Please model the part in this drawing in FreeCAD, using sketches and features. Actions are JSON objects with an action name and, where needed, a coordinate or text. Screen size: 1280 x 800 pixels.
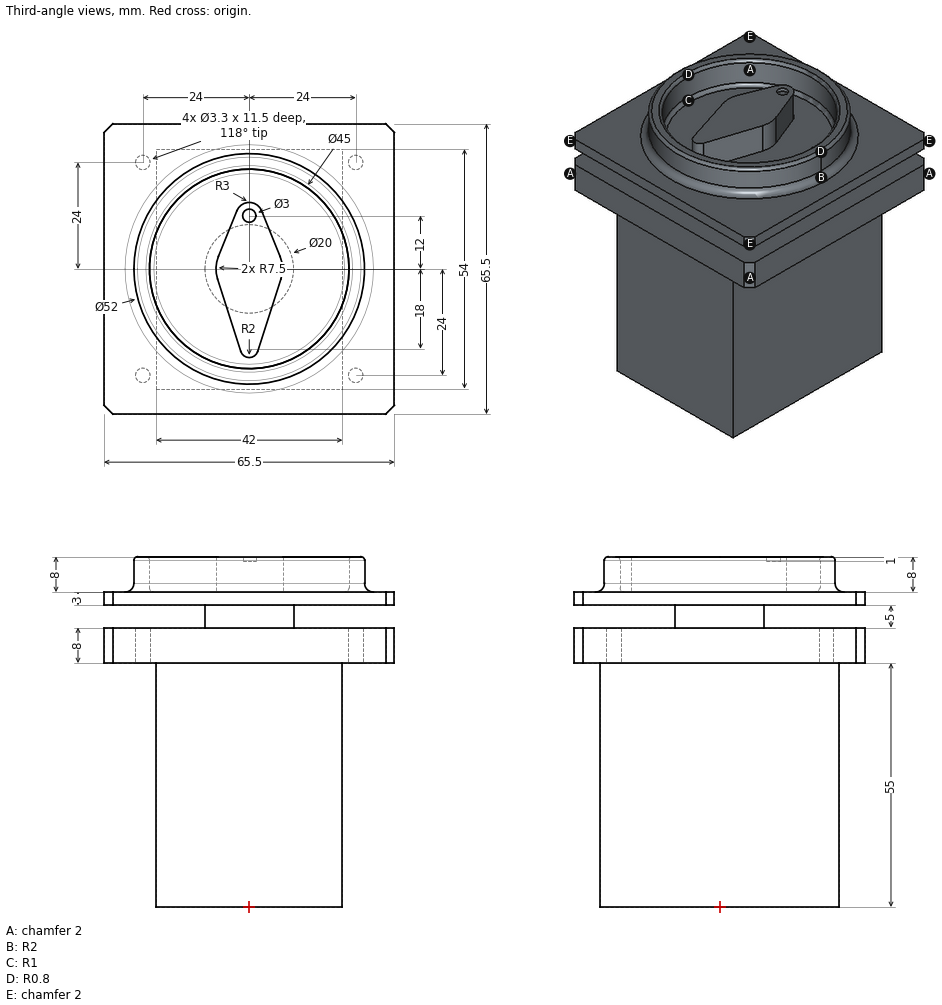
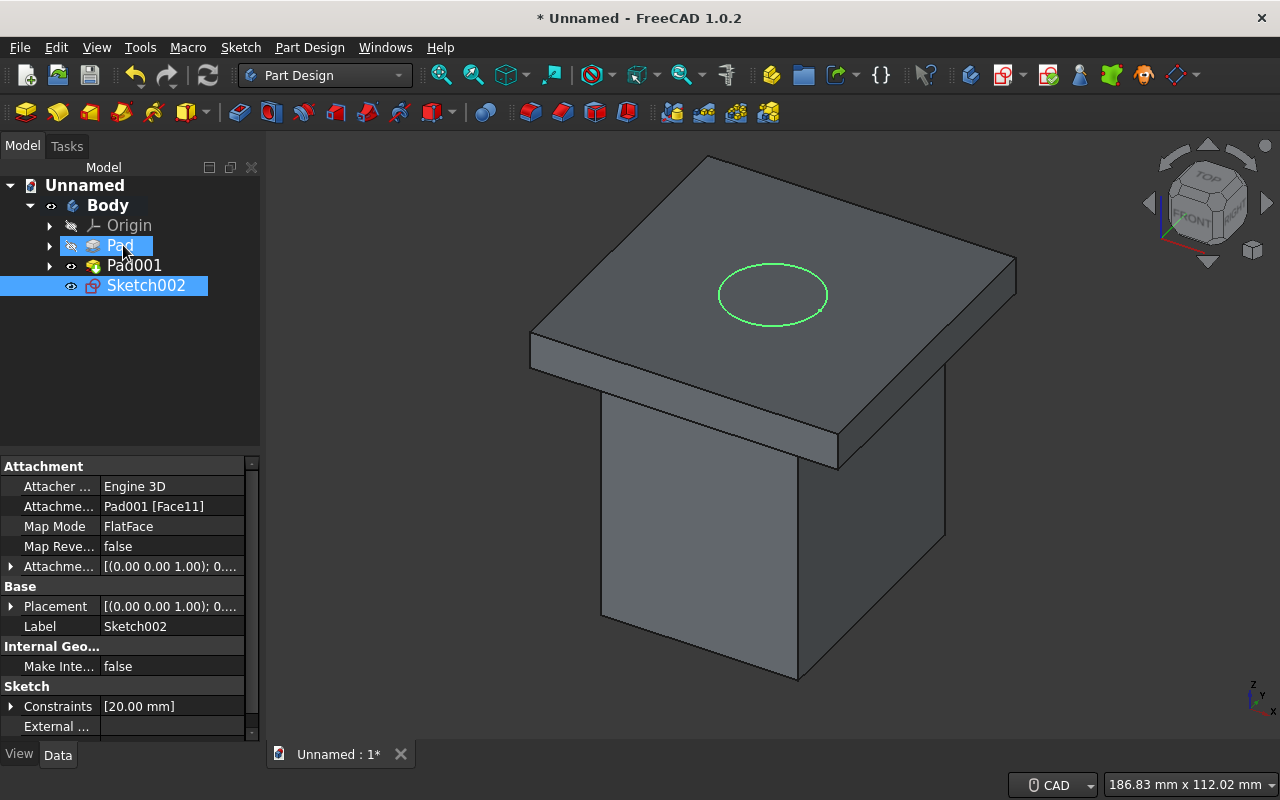
{"action": "left_click", "coordinate": [26, 112]}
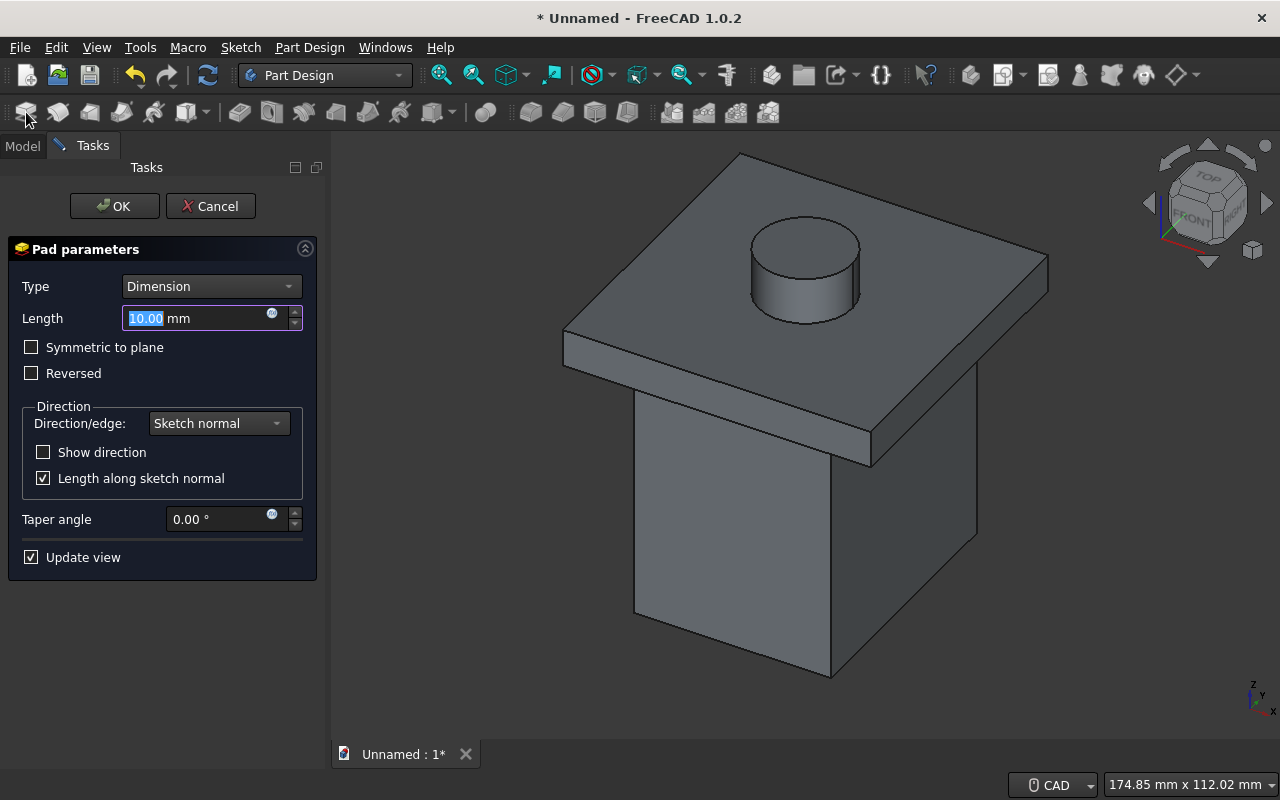
{"action": "type", "text": "5"}
{"action": "key", "text": "Tab"}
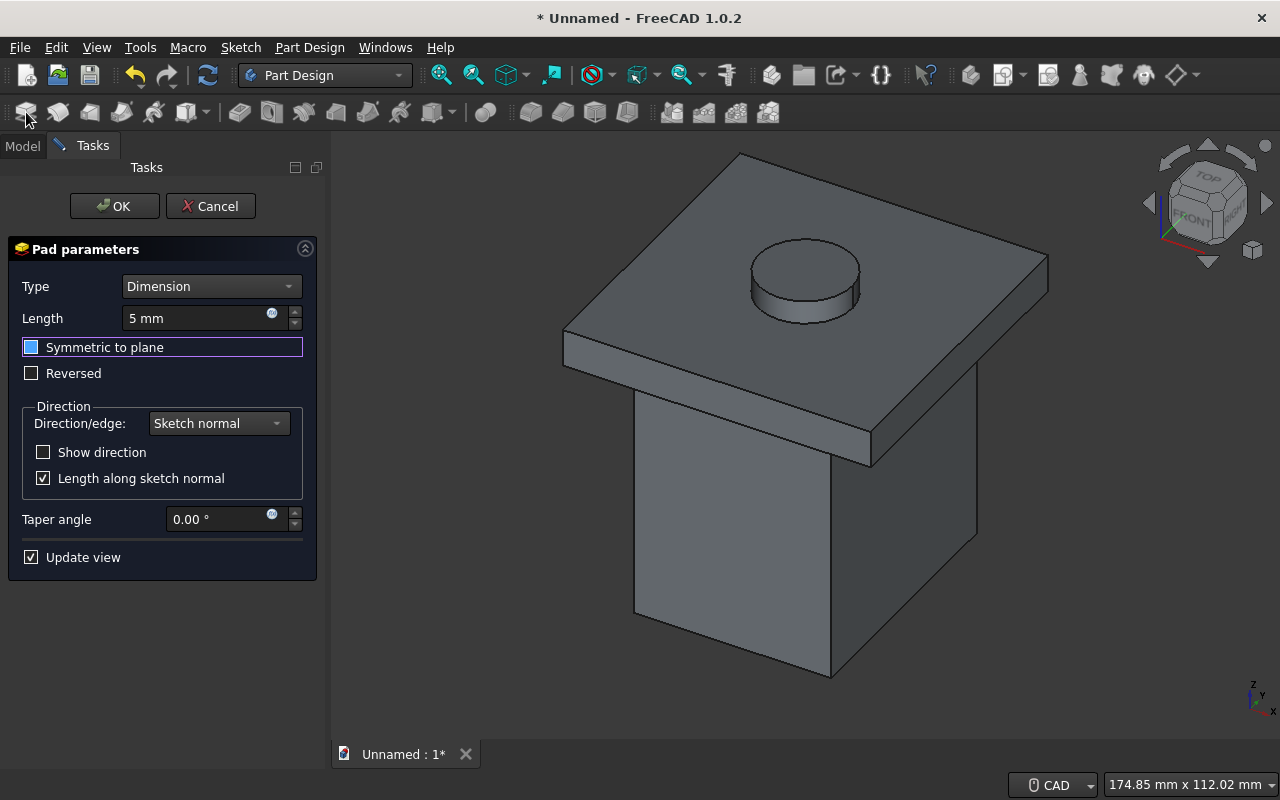
{"action": "left_click", "coordinate": [115, 206]}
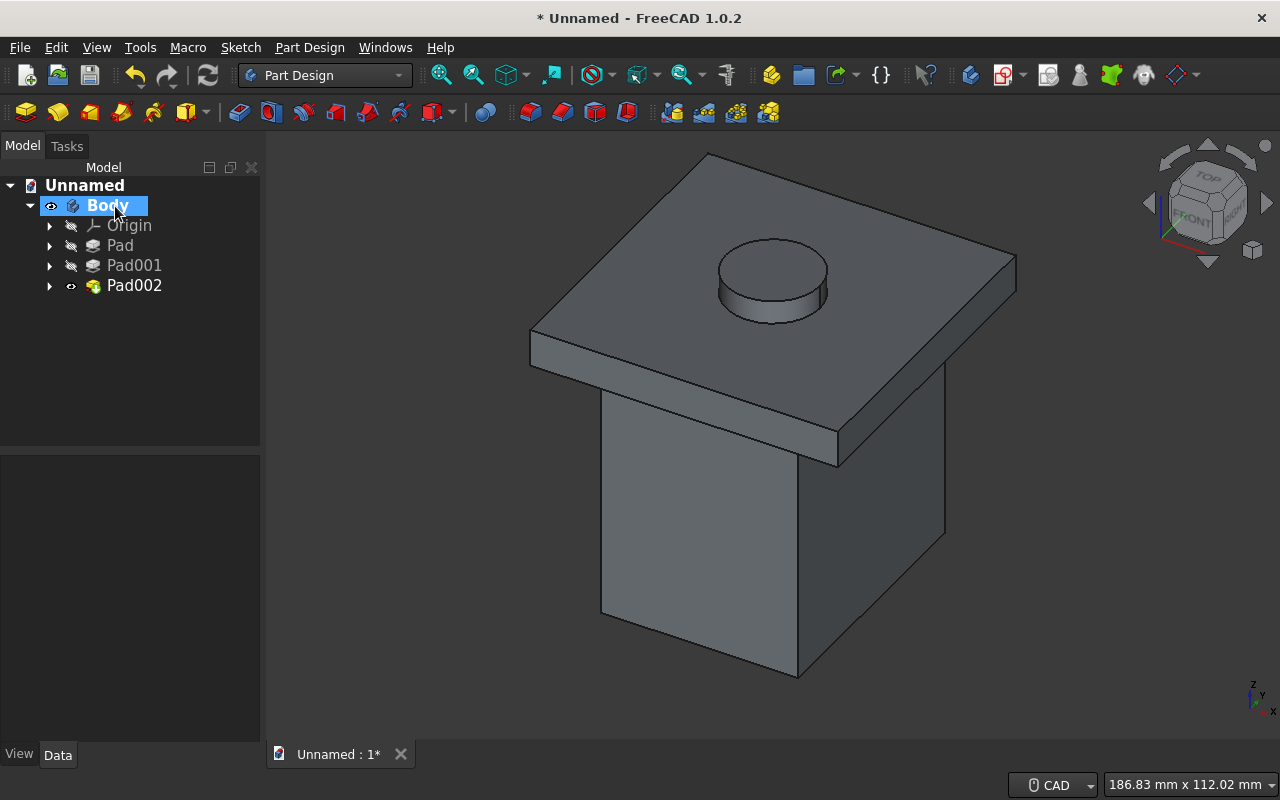
{"action": "left_click", "coordinate": [442, 76]}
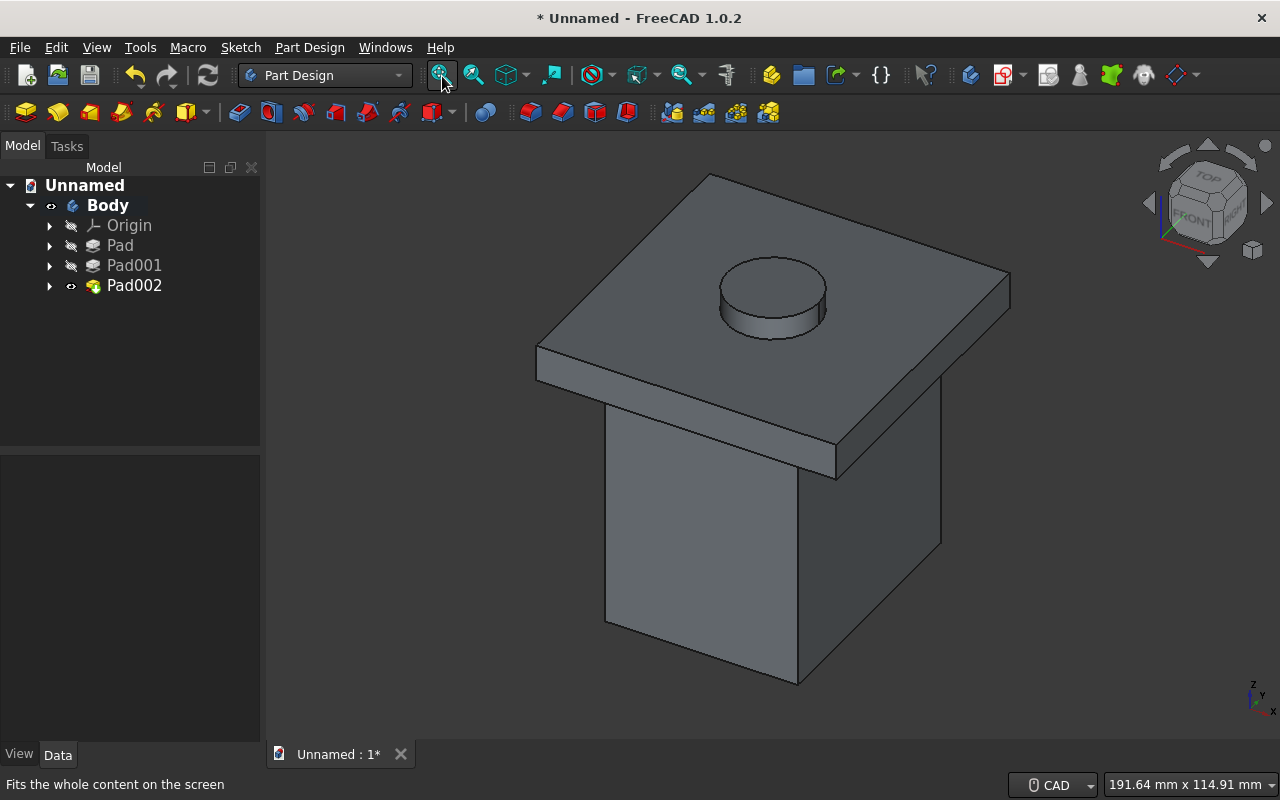
{"action": "left_click", "coordinate": [908, 288]}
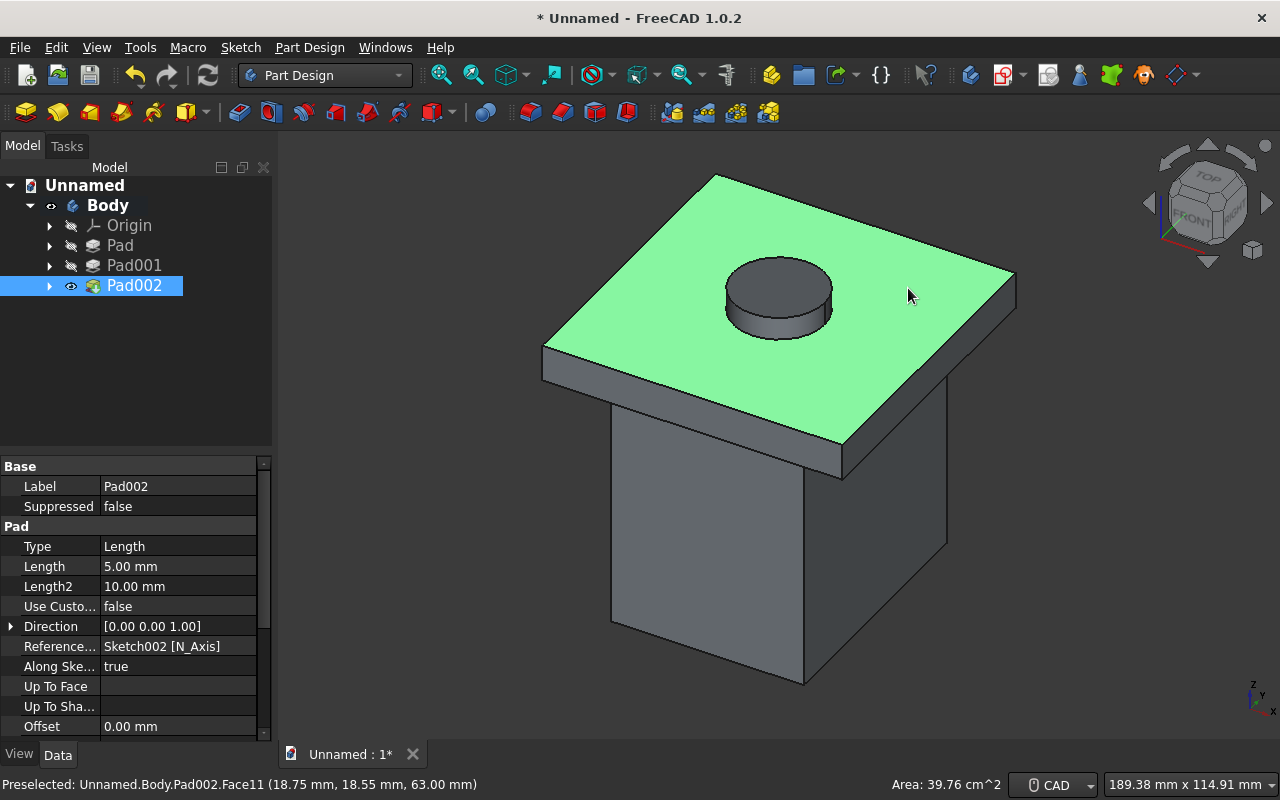
{"action": "left_click", "coordinate": [1004, 76]}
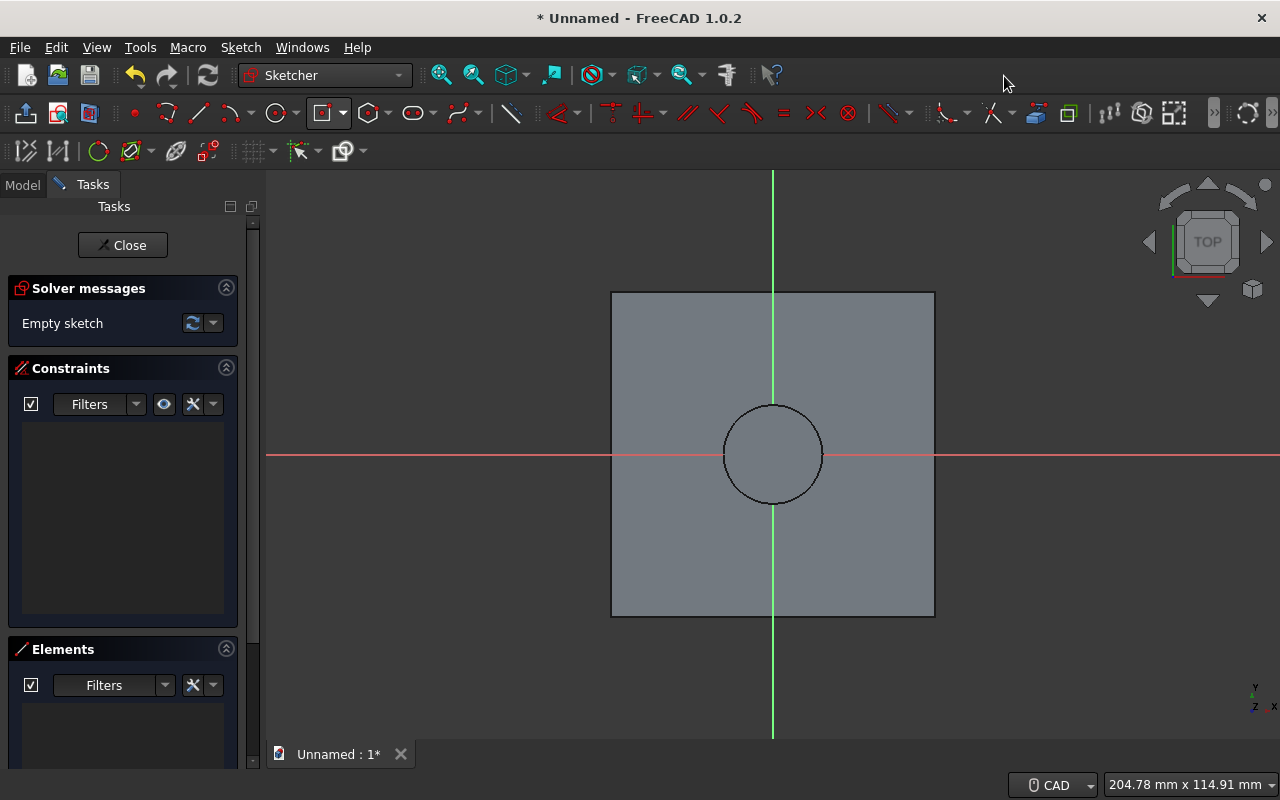
{"action": "left_click", "coordinate": [90, 114]}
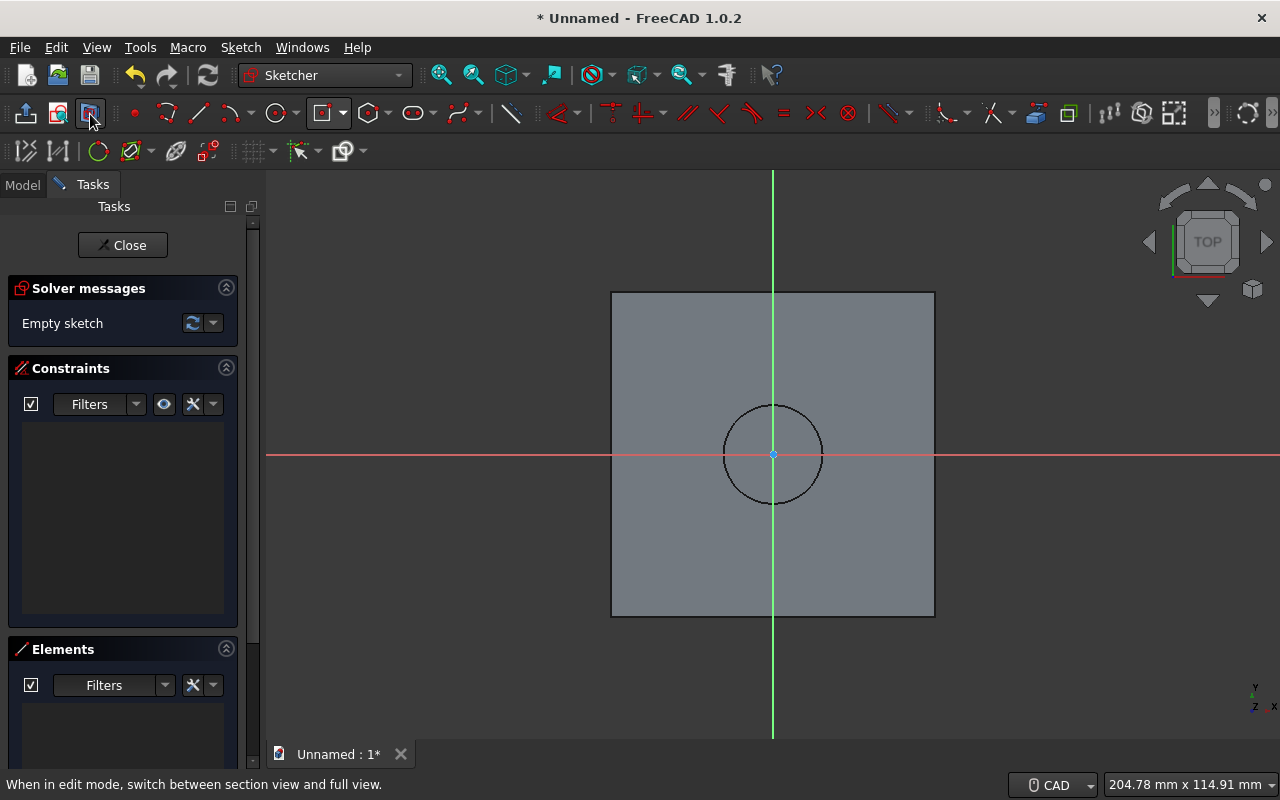
{"action": "scroll", "coordinate": [912, 455], "scroll_direction": "up", "scroll_amount": 2}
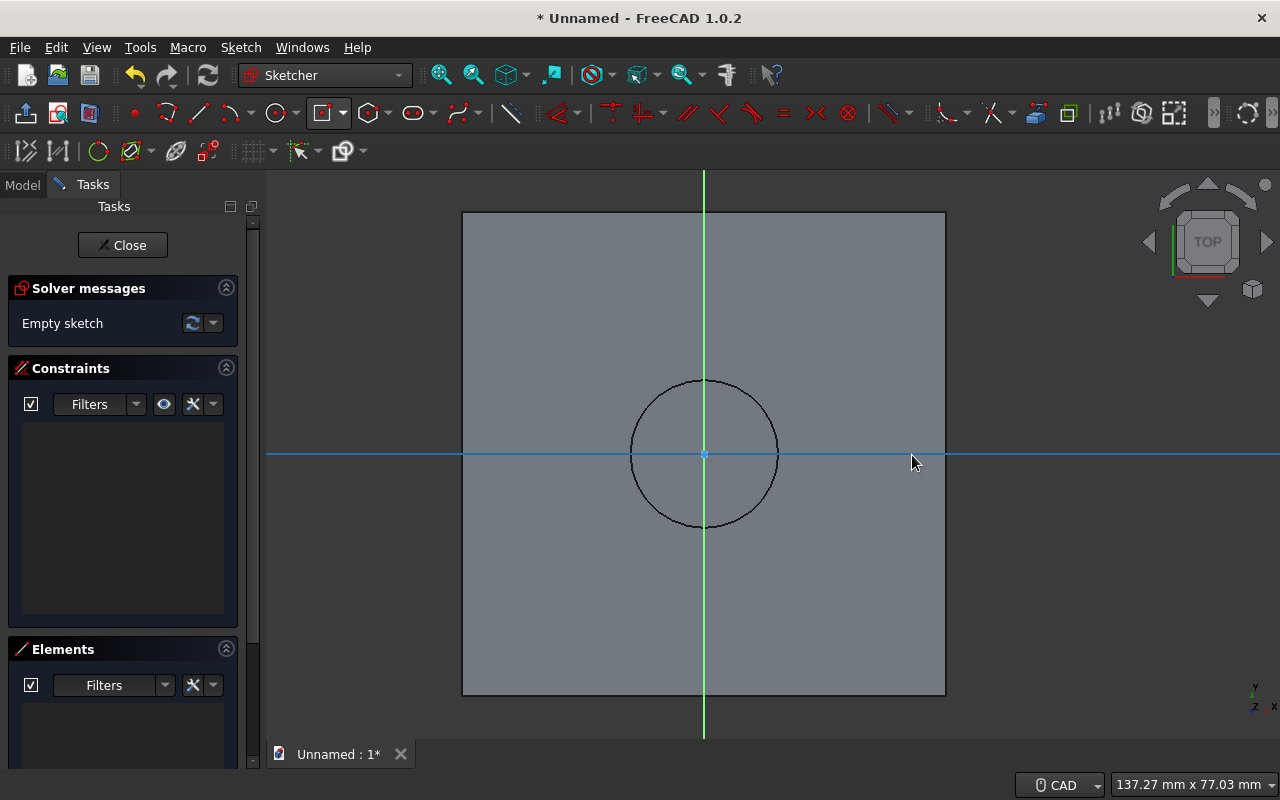
{"action": "left_click", "coordinate": [276, 114]}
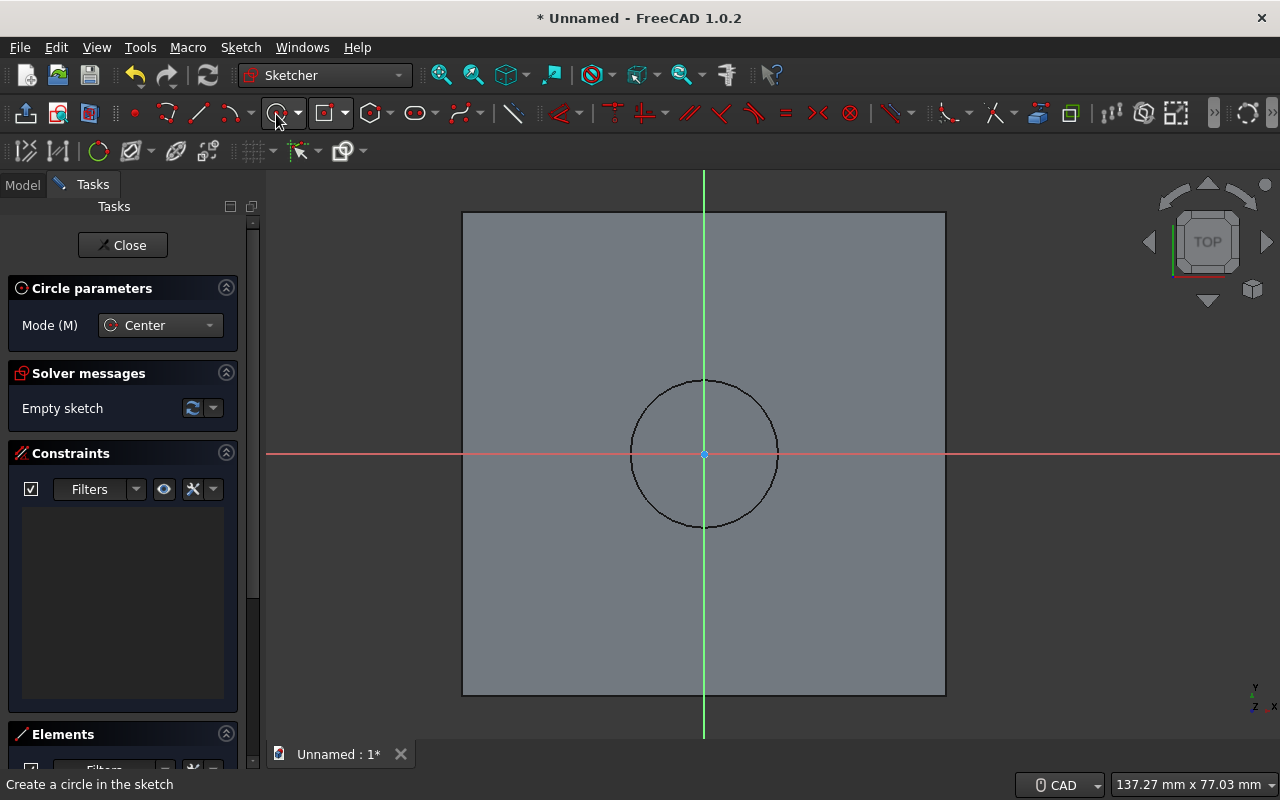
{"action": "scroll", "coordinate": [527, 277], "scroll_direction": "up", "scroll_amount": 4}